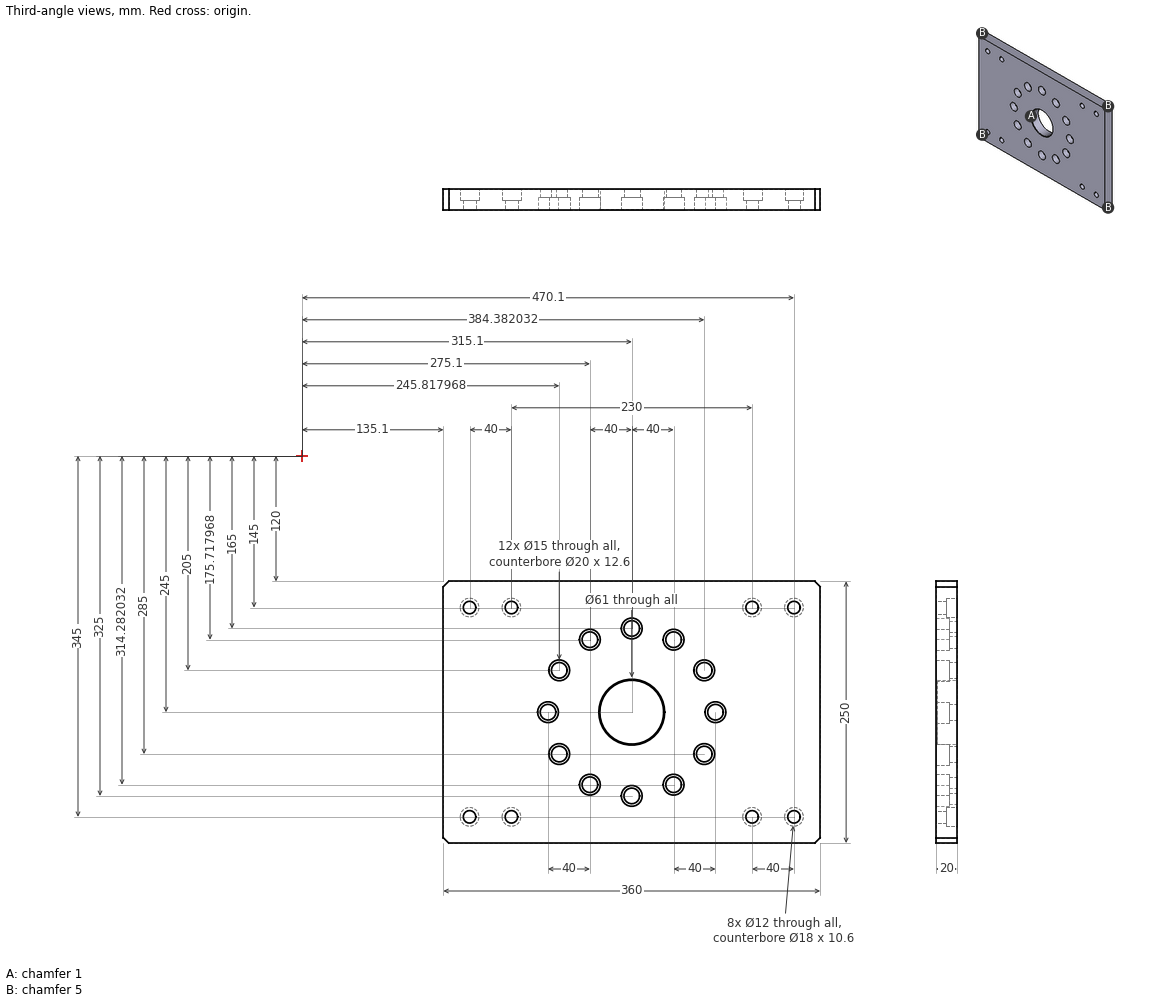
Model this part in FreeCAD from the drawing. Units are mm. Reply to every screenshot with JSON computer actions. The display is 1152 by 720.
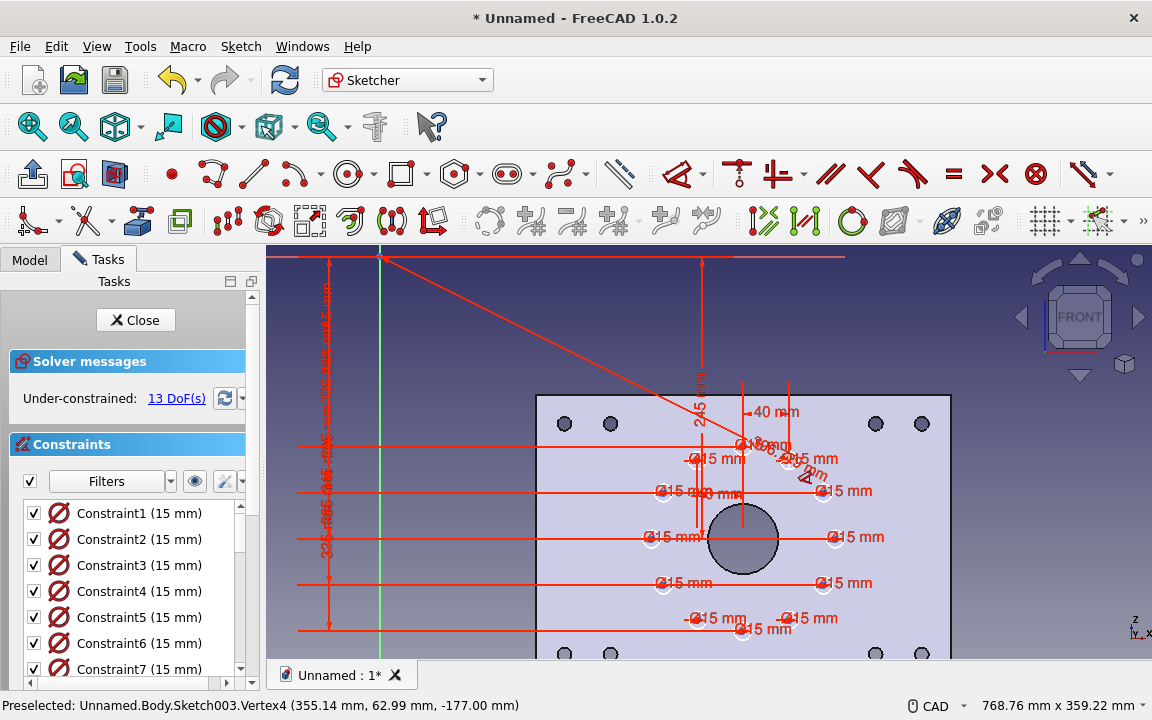
{"action": "left_click", "coordinate": [835, 539]}
{"action": "left_click", "coordinate": [802, 573]}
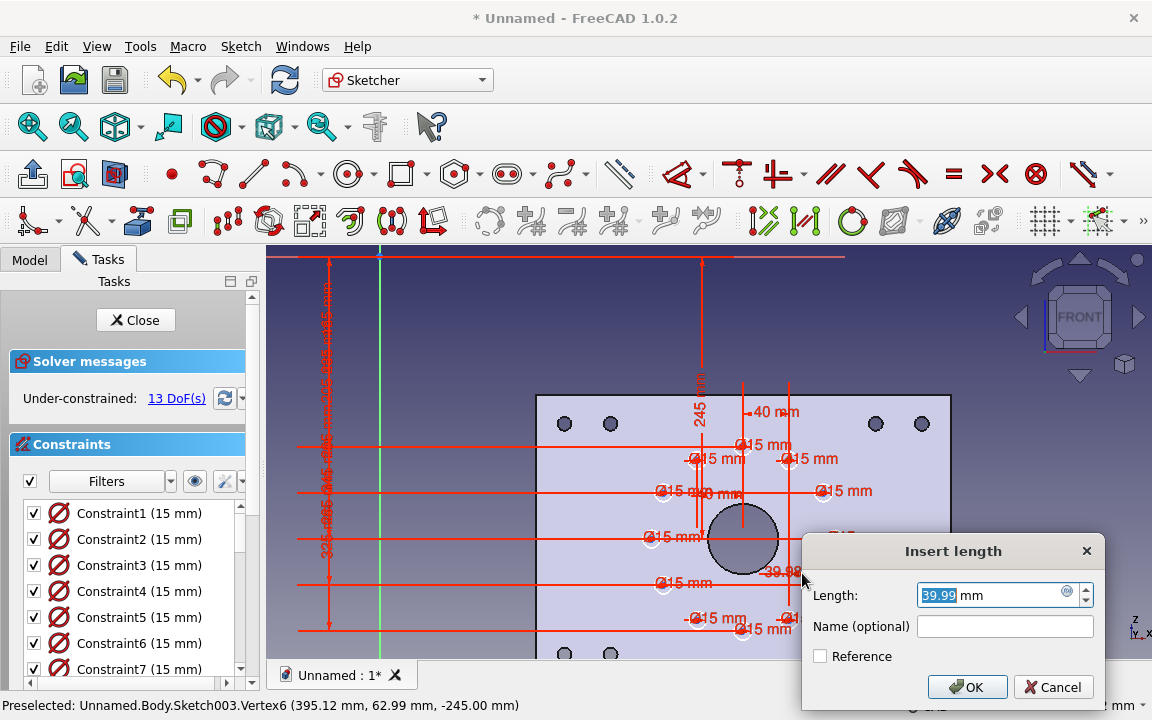
{"action": "type", "text": "40"}
{"action": "key", "text": "Return"}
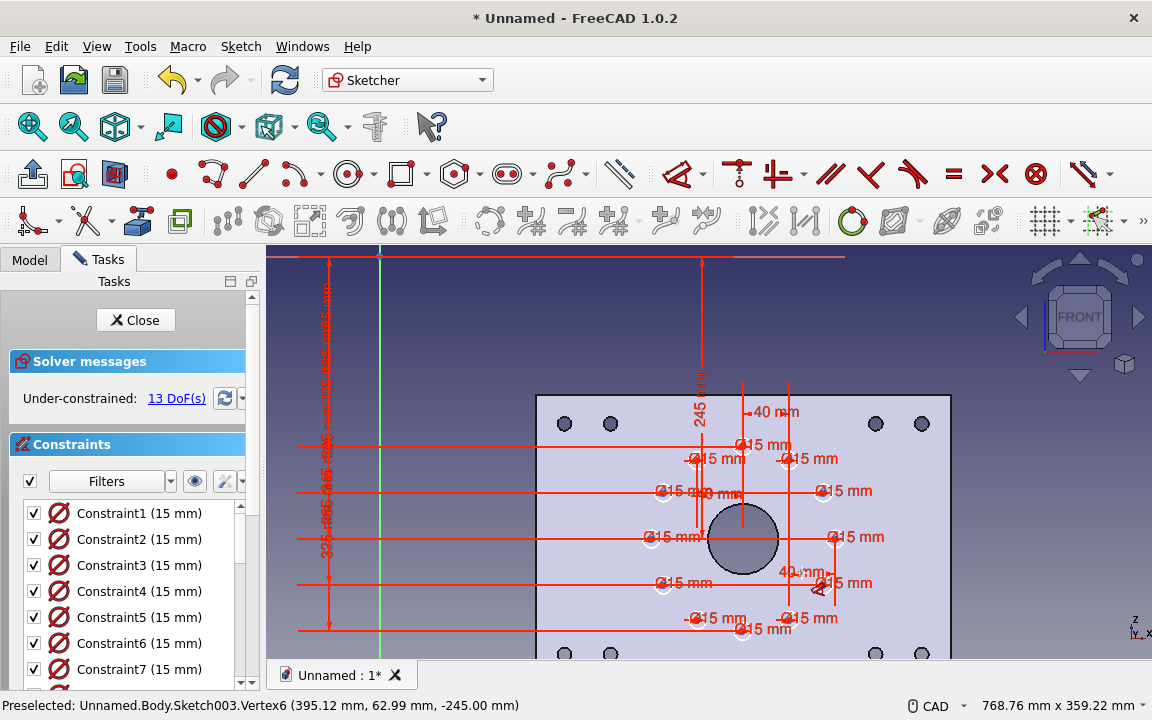
{"action": "left_click", "coordinate": [835, 539]}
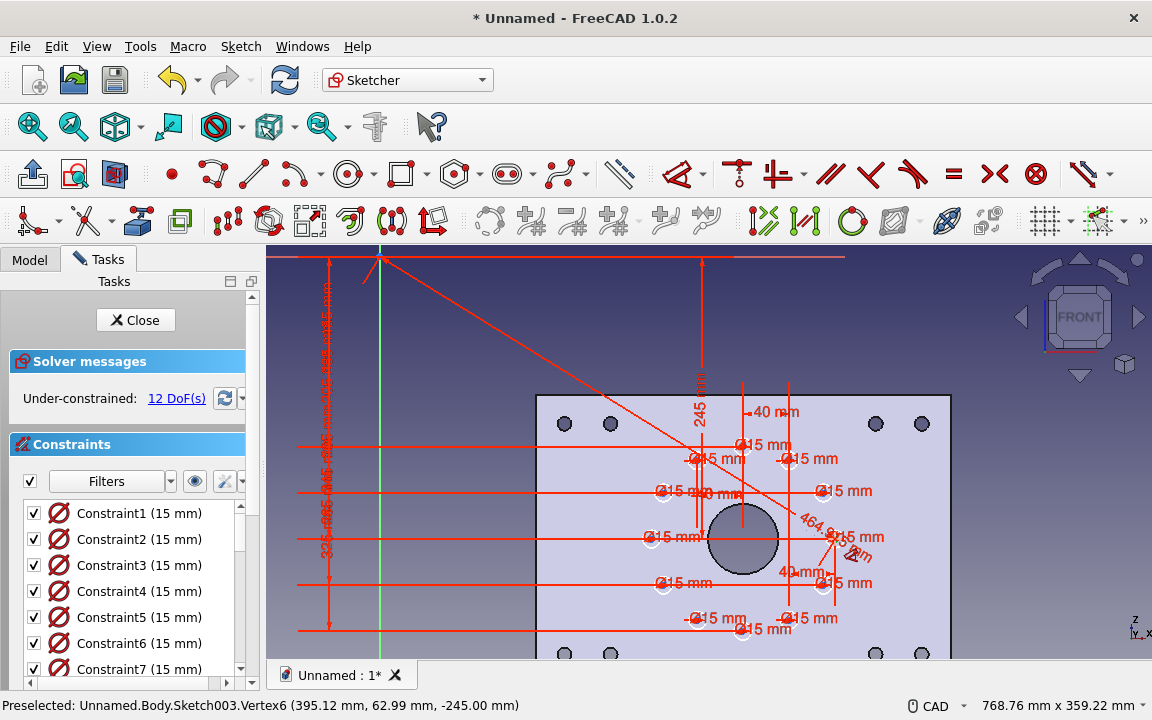
{"action": "left_click", "coordinate": [789, 620]}
{"action": "left_click", "coordinate": [802, 505]}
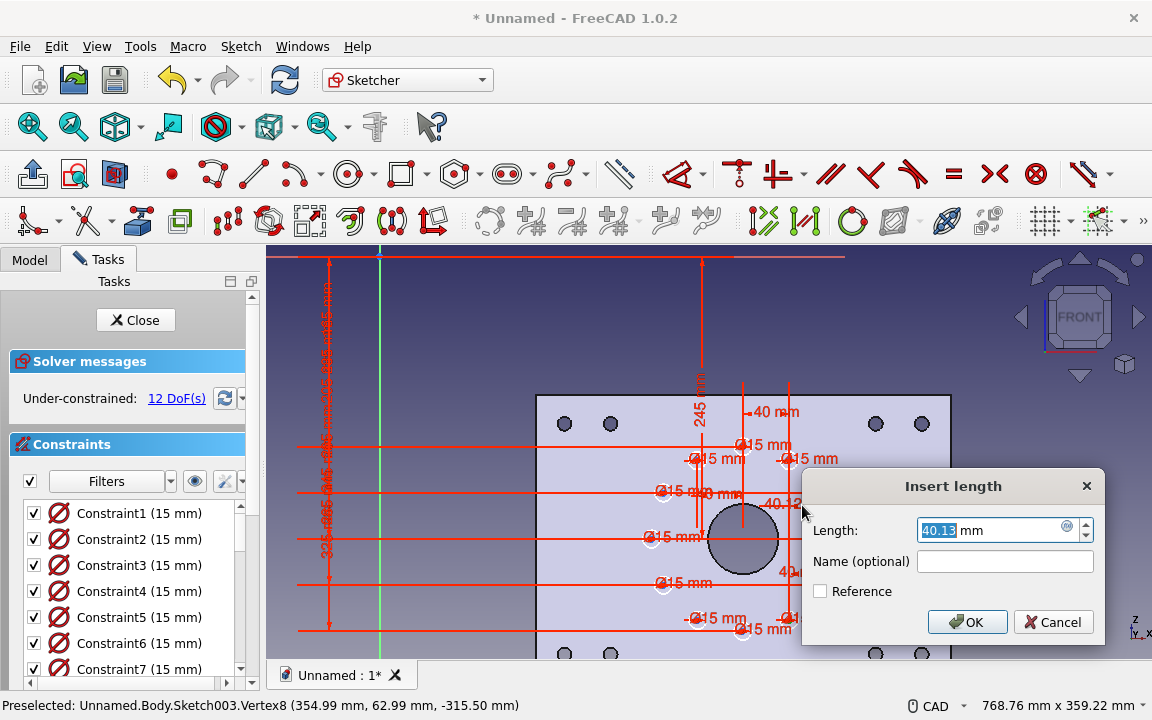
{"action": "type", "text": "40"}
{"action": "key", "text": "Return"}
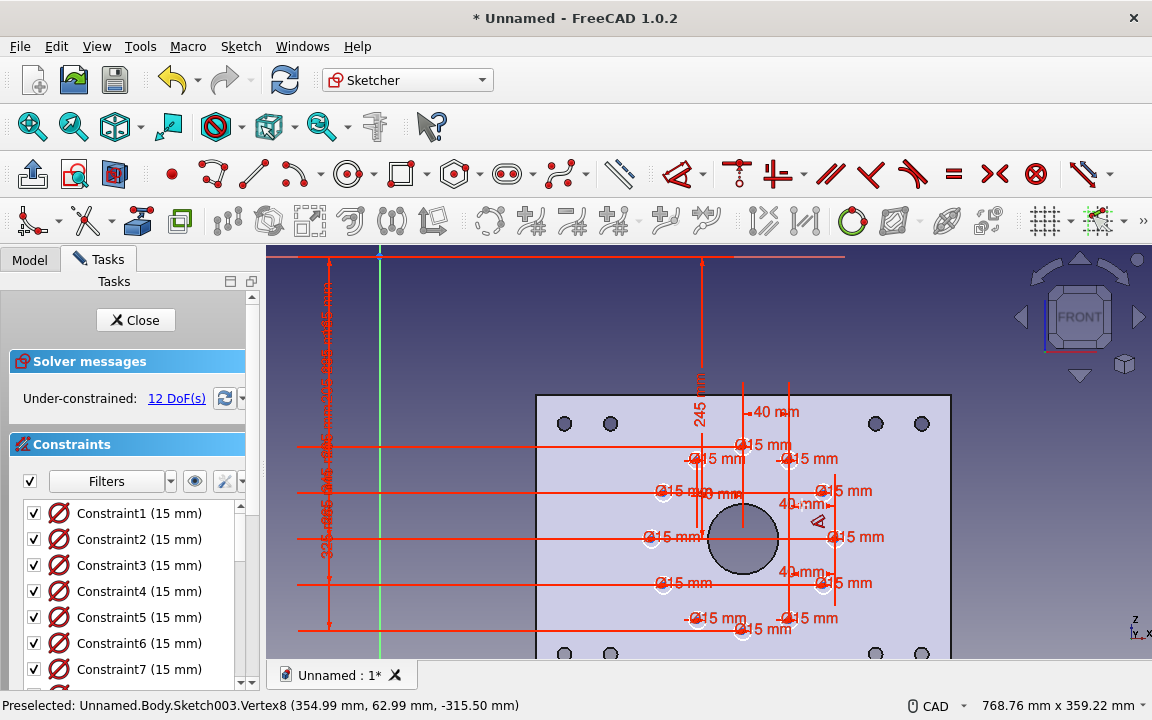
{"action": "left_click", "coordinate": [789, 620]}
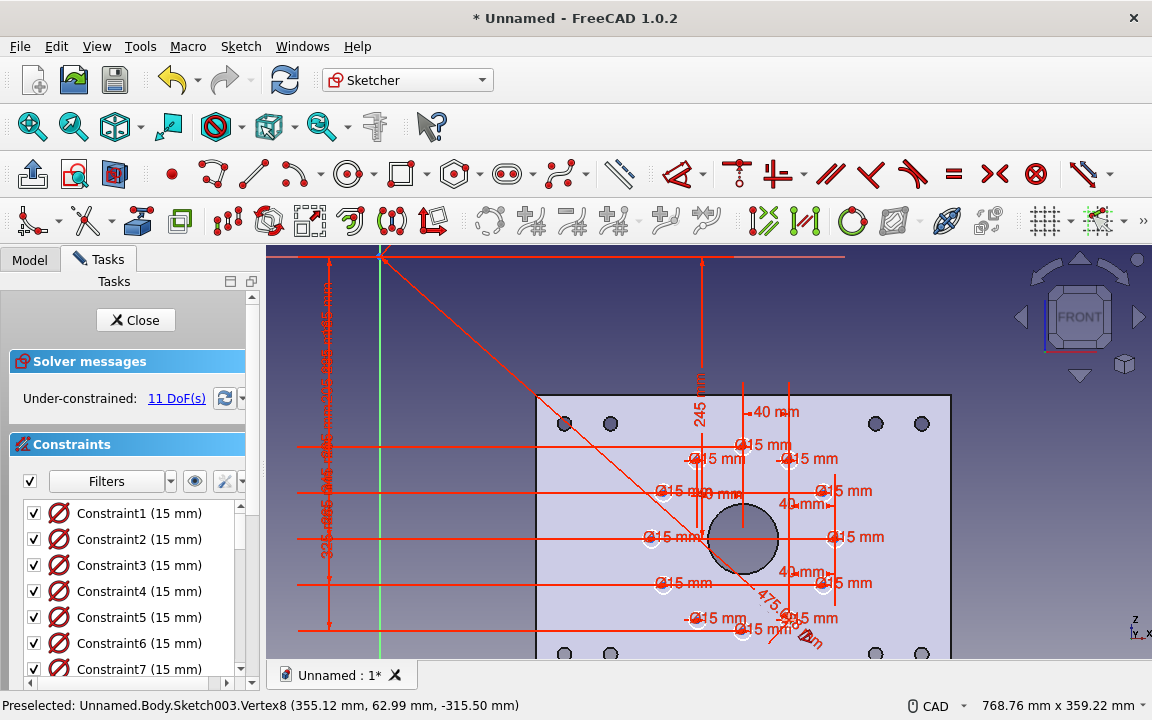
{"action": "scroll", "coordinate": [698, 459], "scroll_direction": "down", "scroll_amount": 2}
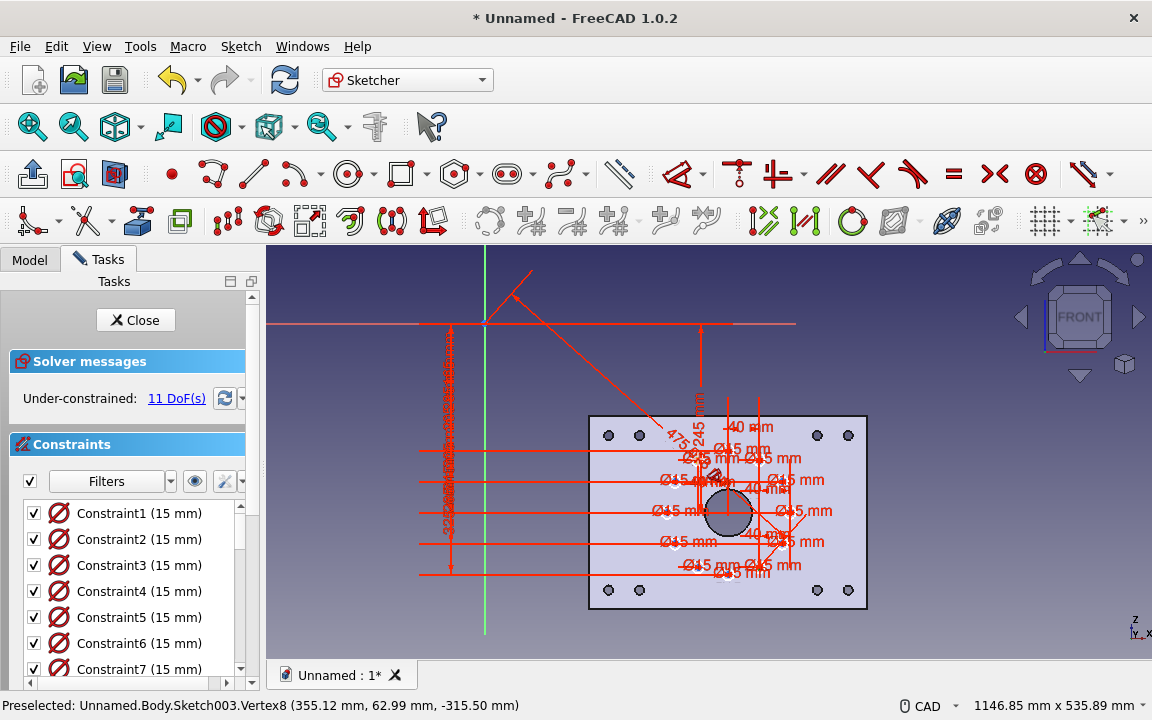
{"action": "scroll", "coordinate": [728, 575], "scroll_direction": "up", "scroll_amount": 2}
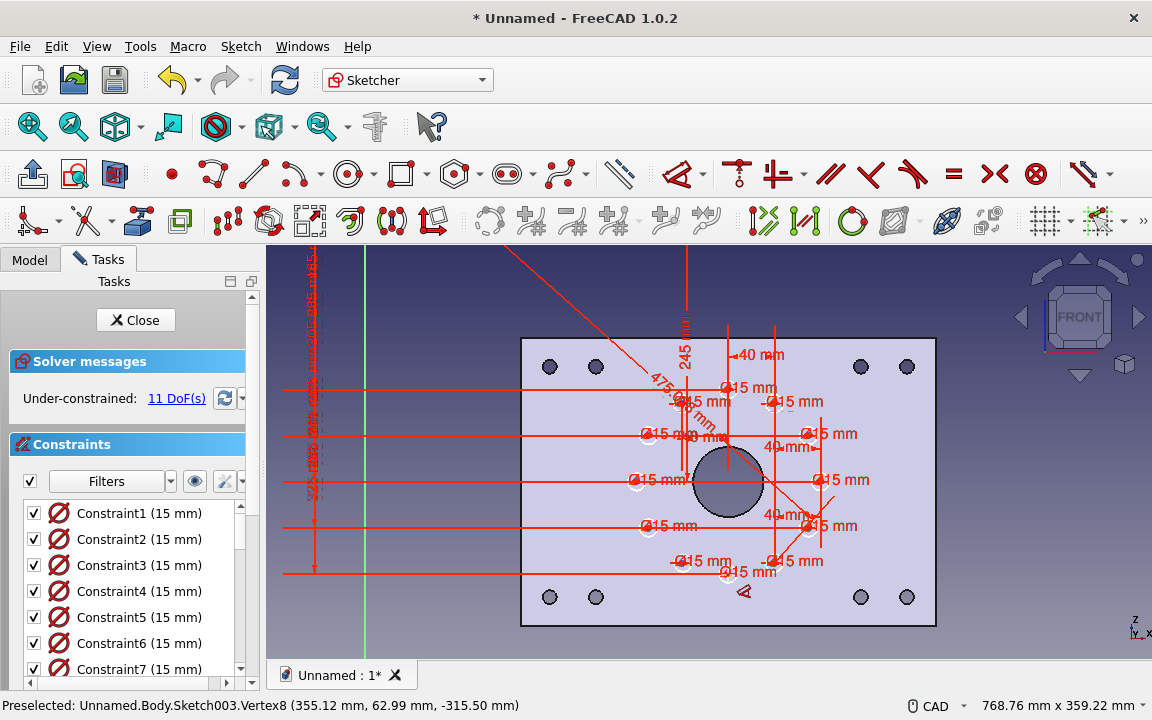
{"action": "left_click", "coordinate": [728, 574]}
{"action": "left_click", "coordinate": [751, 608]}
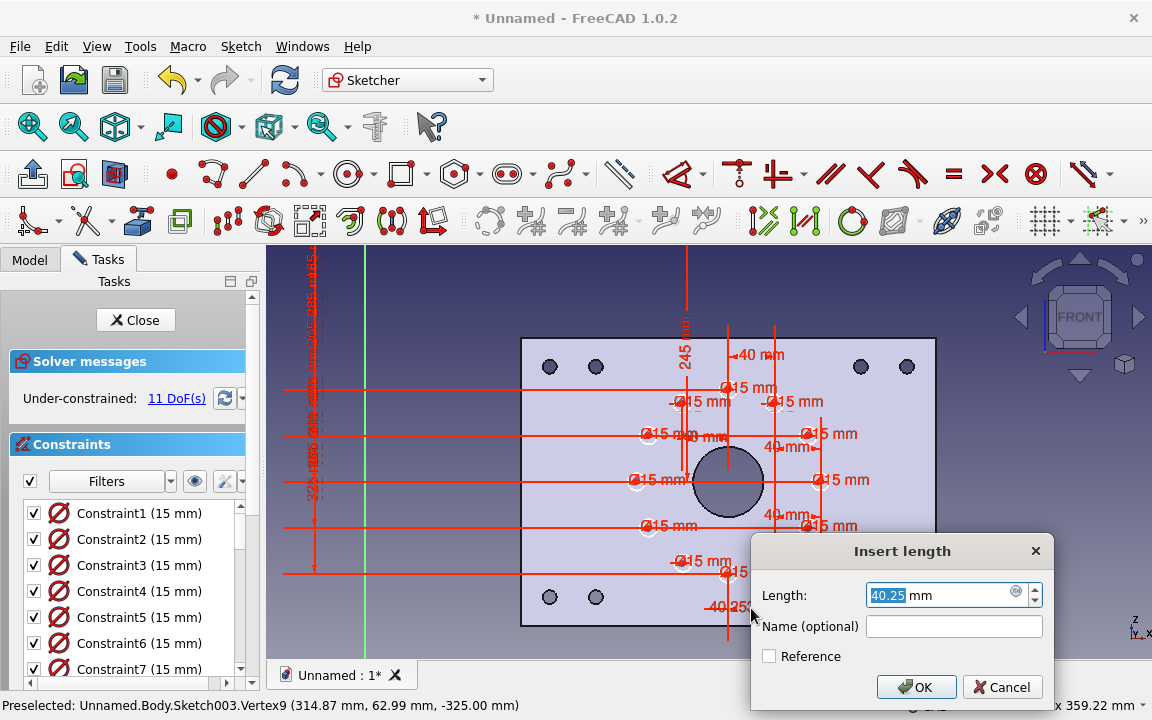
{"action": "type", "text": "40"}
{"action": "key", "text": "Return"}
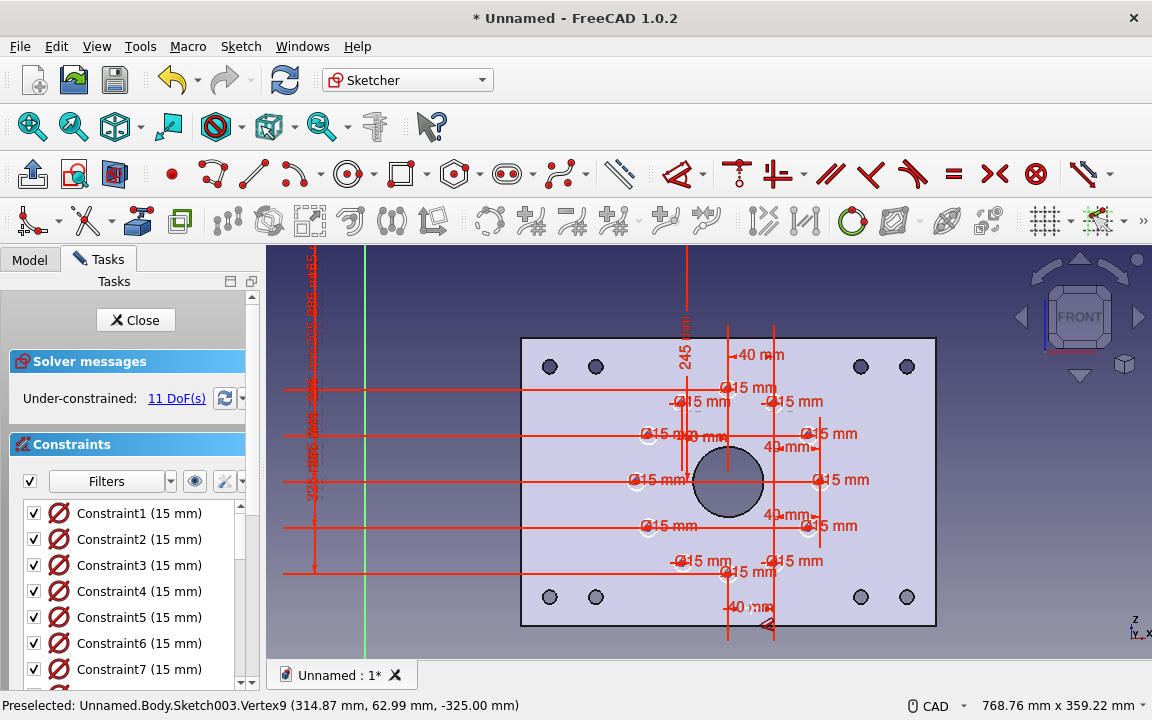
{"action": "left_click", "coordinate": [728, 574]}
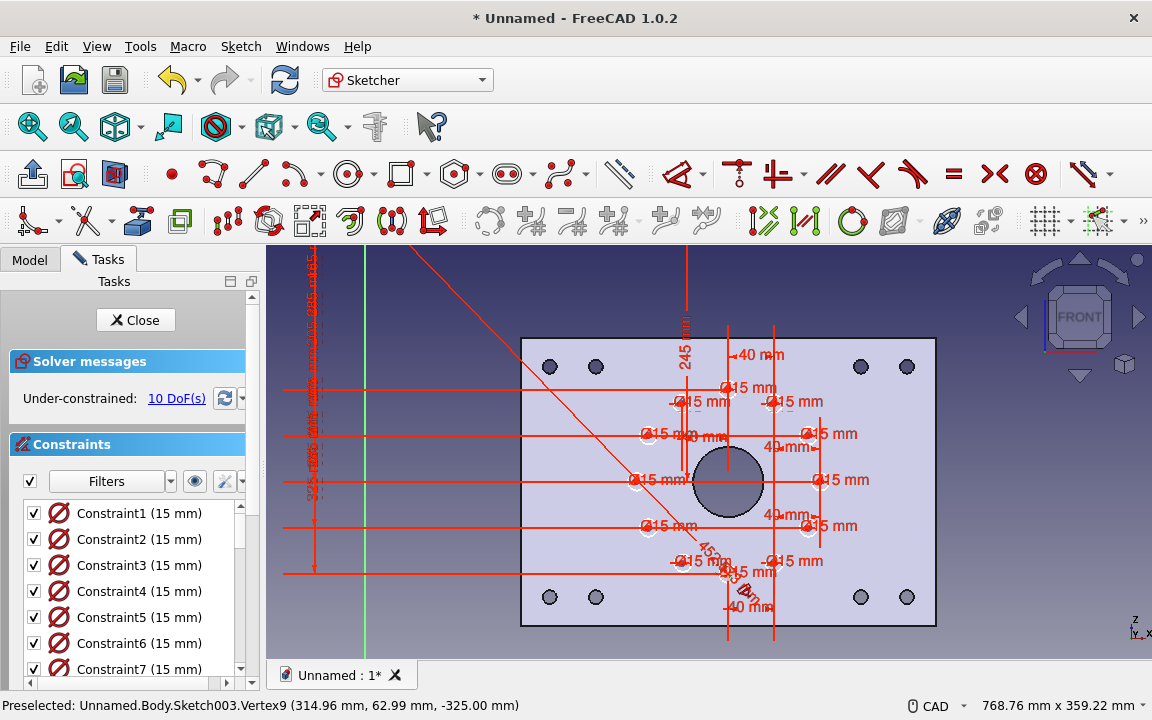
{"action": "left_click", "coordinate": [683, 563]}
{"action": "left_click", "coordinate": [706, 529]}